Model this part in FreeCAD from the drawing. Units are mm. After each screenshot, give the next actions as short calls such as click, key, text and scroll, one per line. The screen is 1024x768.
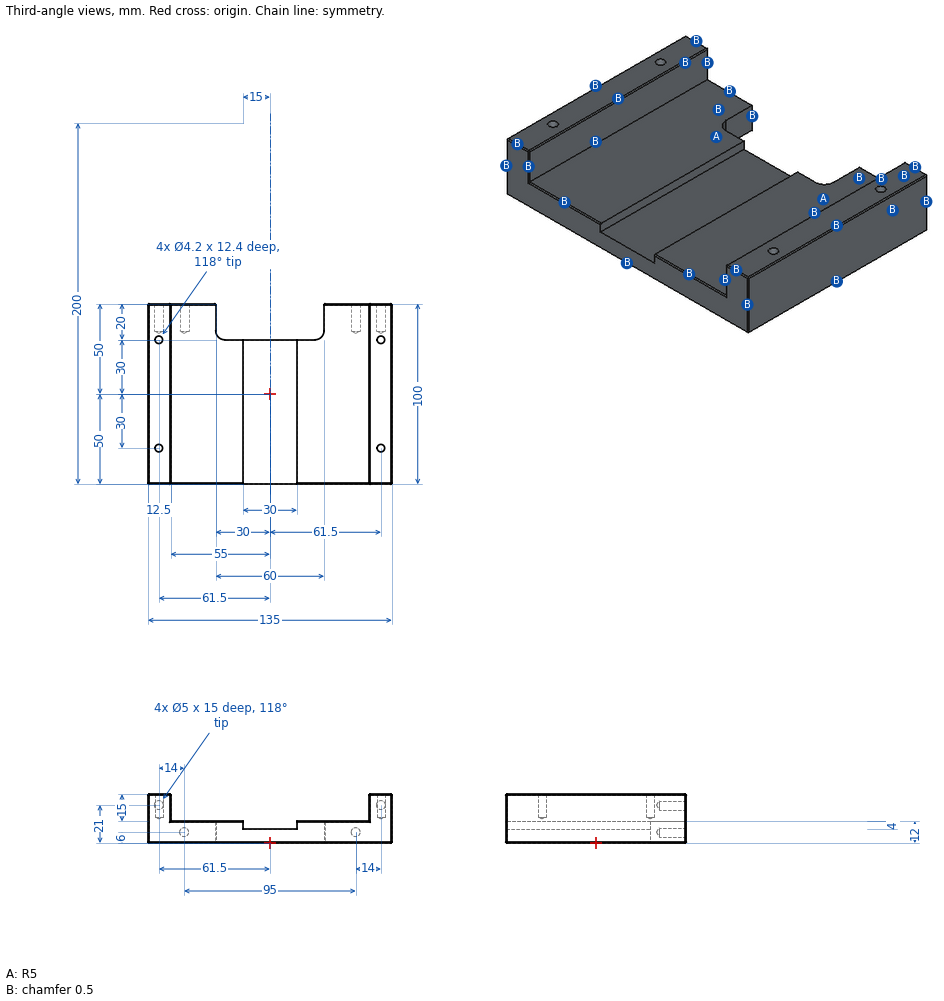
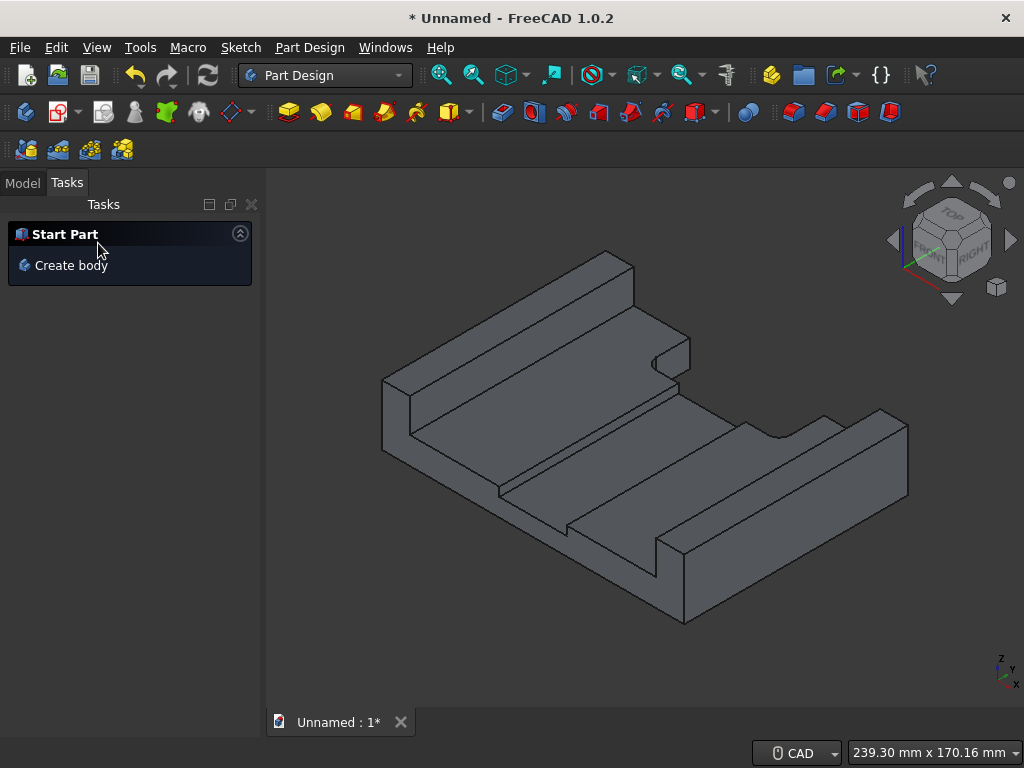
key(4)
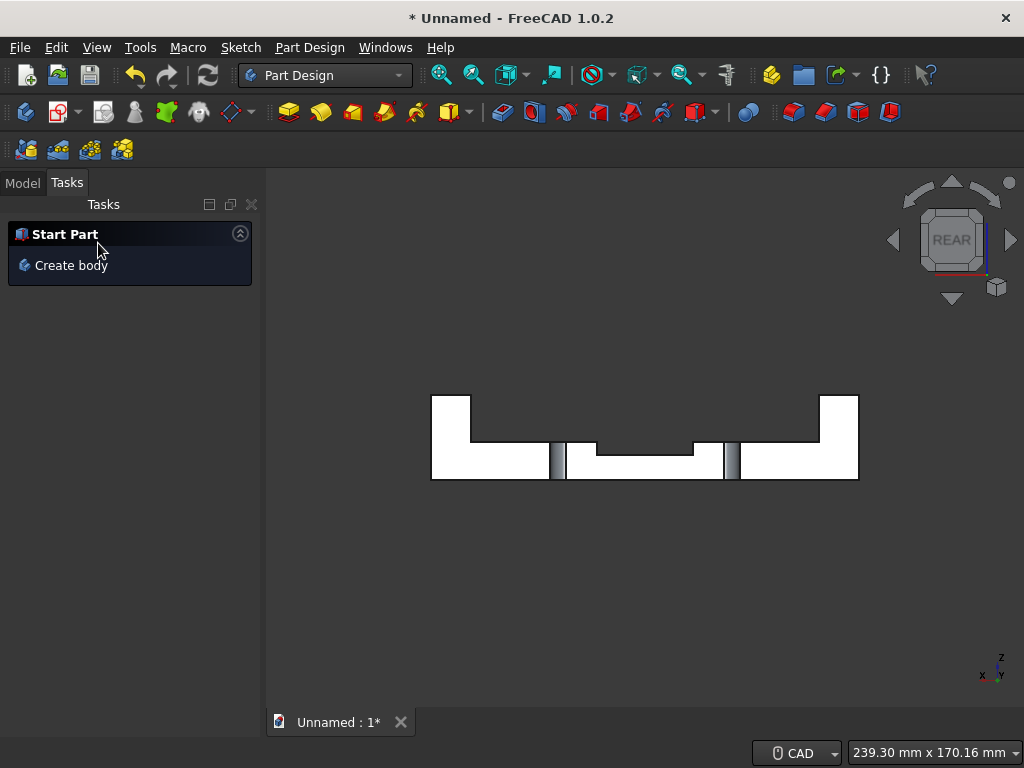
click(765, 461)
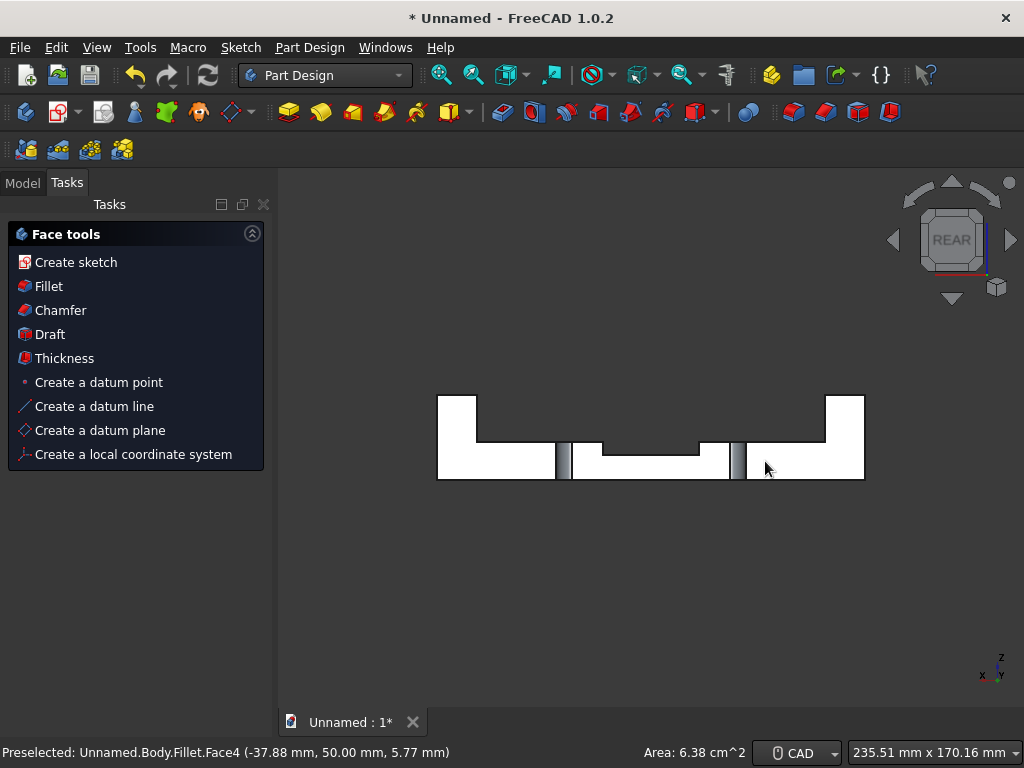
click(58, 112)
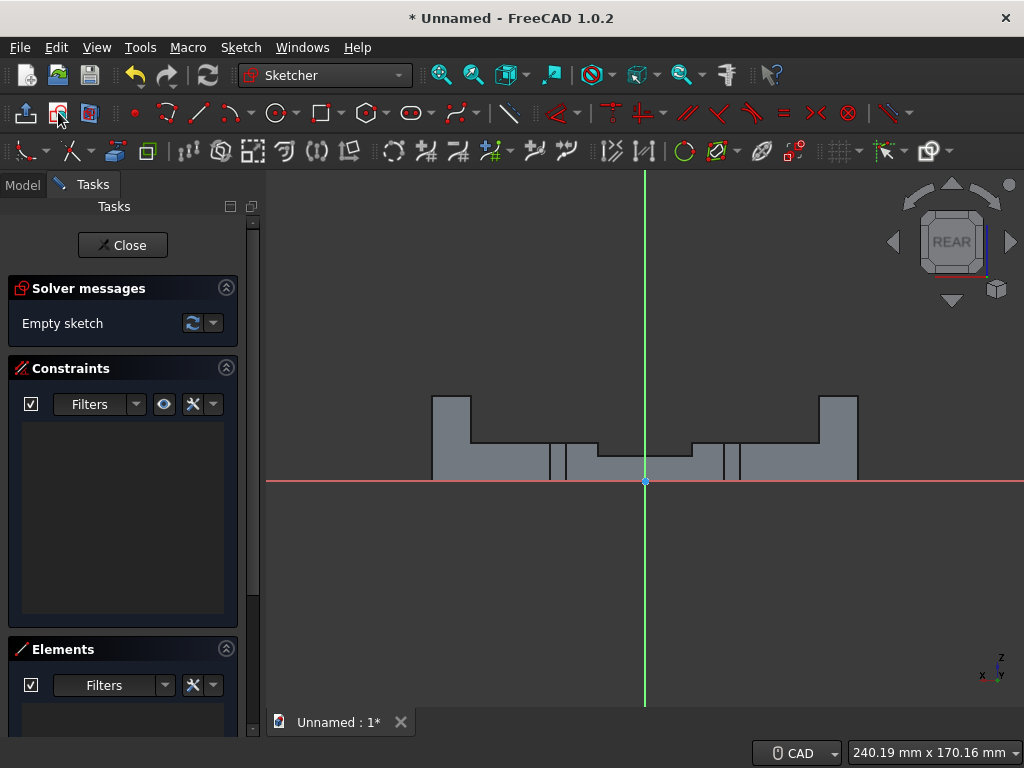
scroll(294, 414, down, 1)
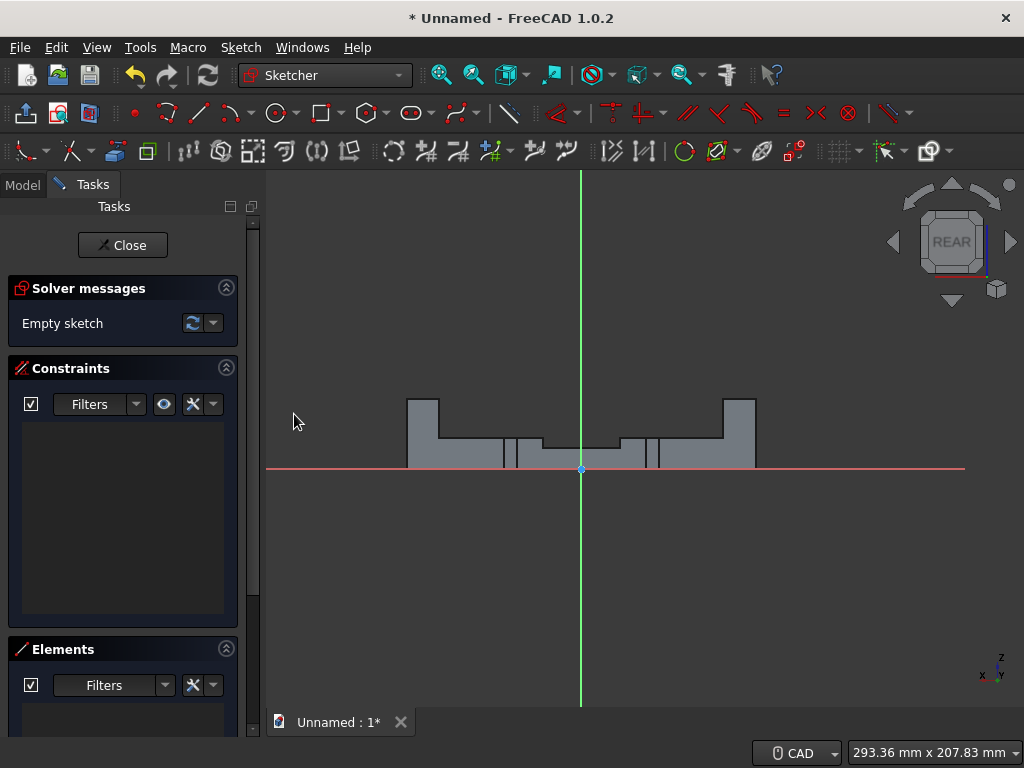
key(g)
key(c)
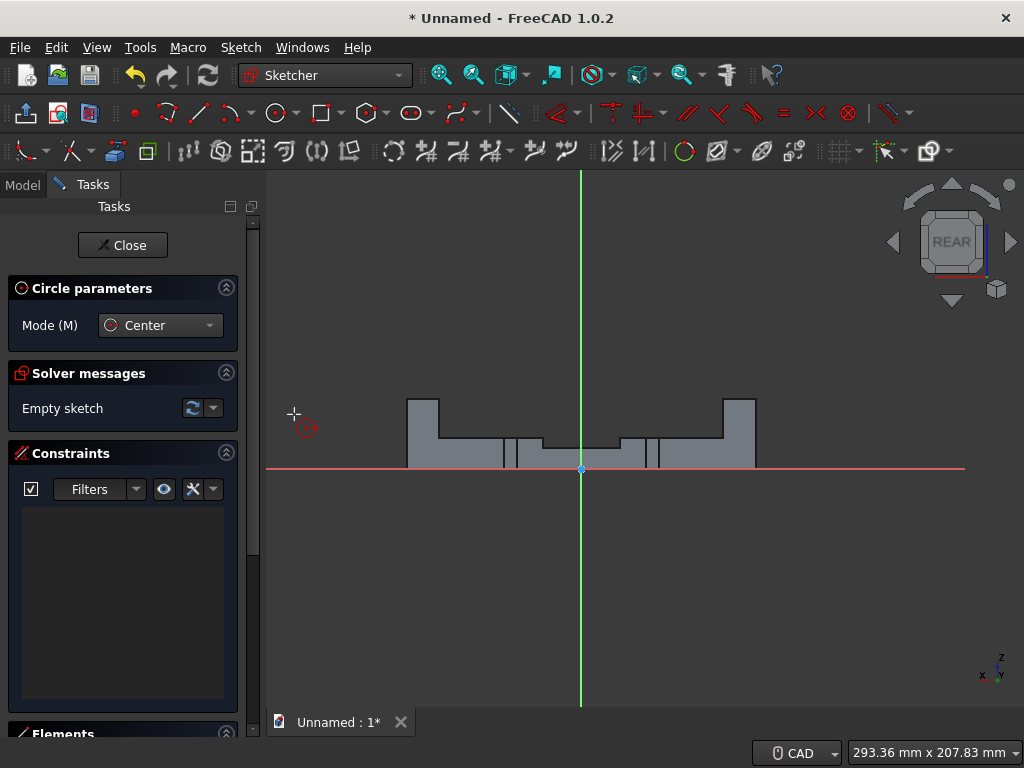
scroll(740, 415, up, 7)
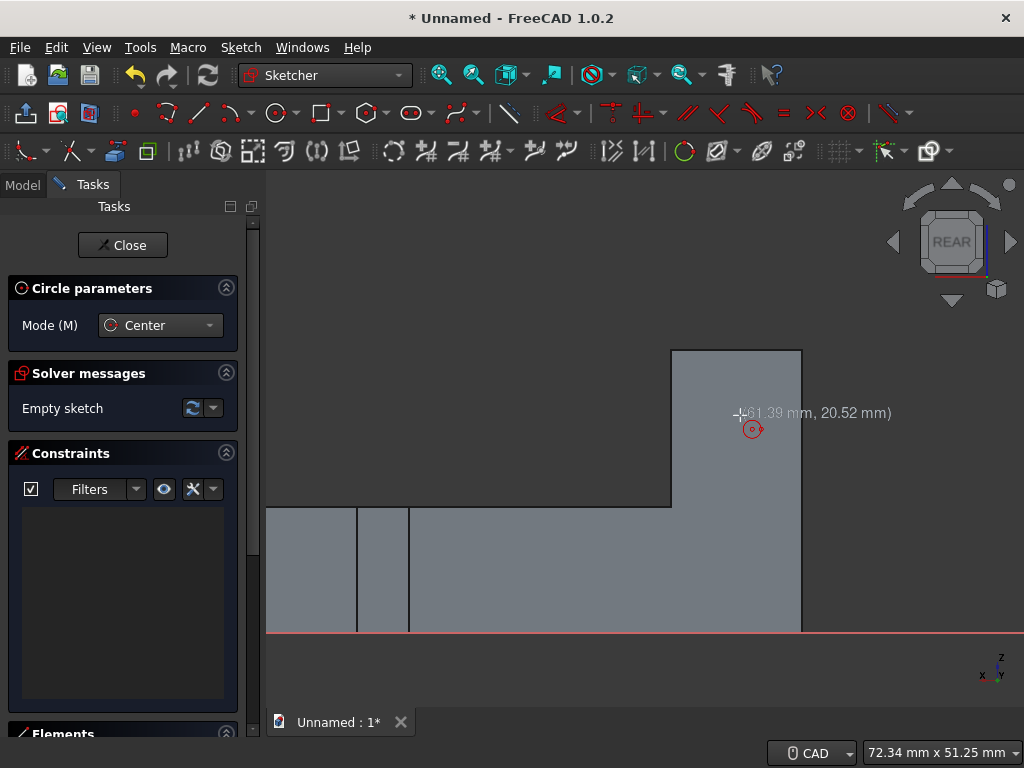
scroll(784, 408, down, 6)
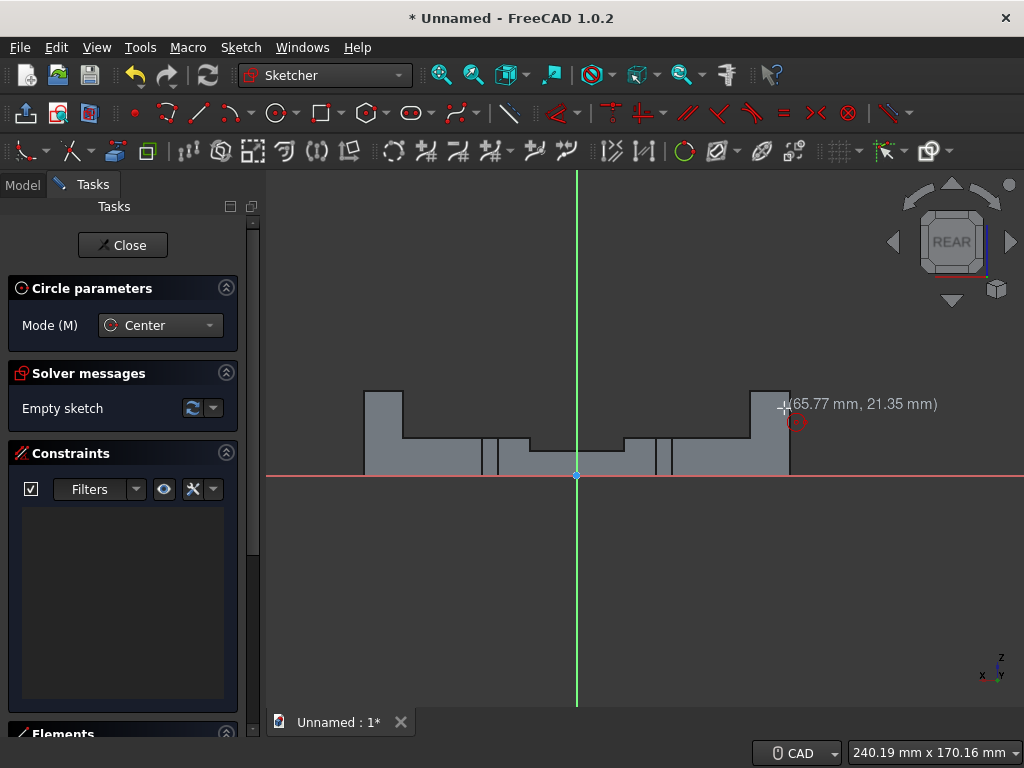
click(771, 410)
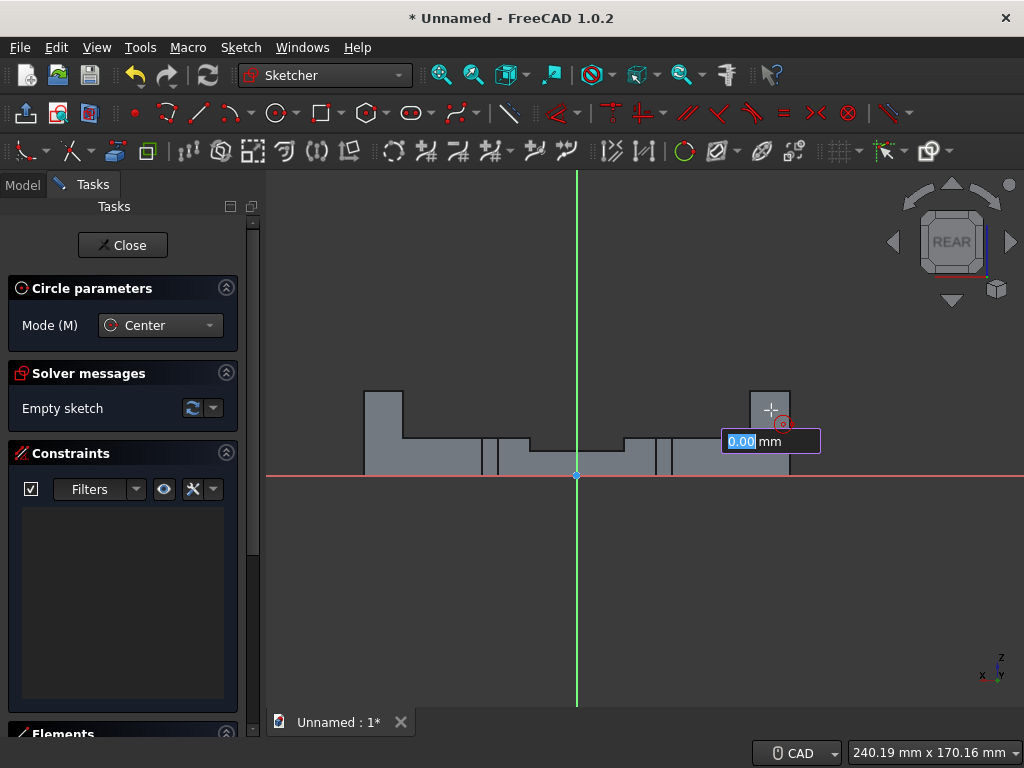
scroll(777, 404, up, 4)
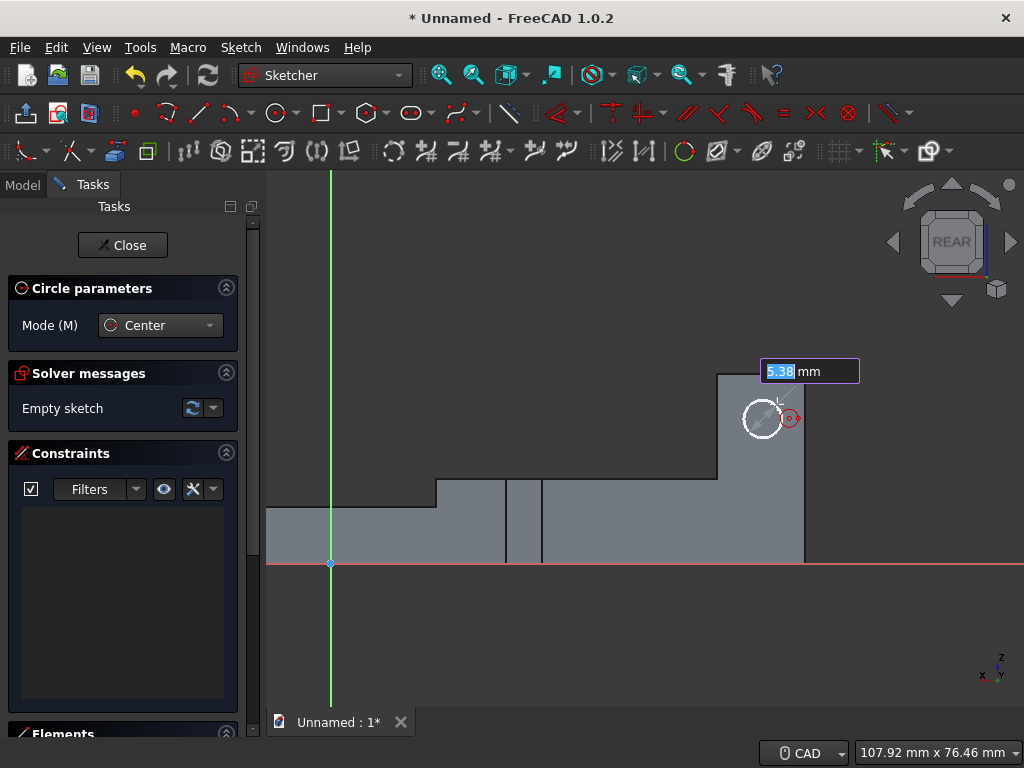
click(775, 404)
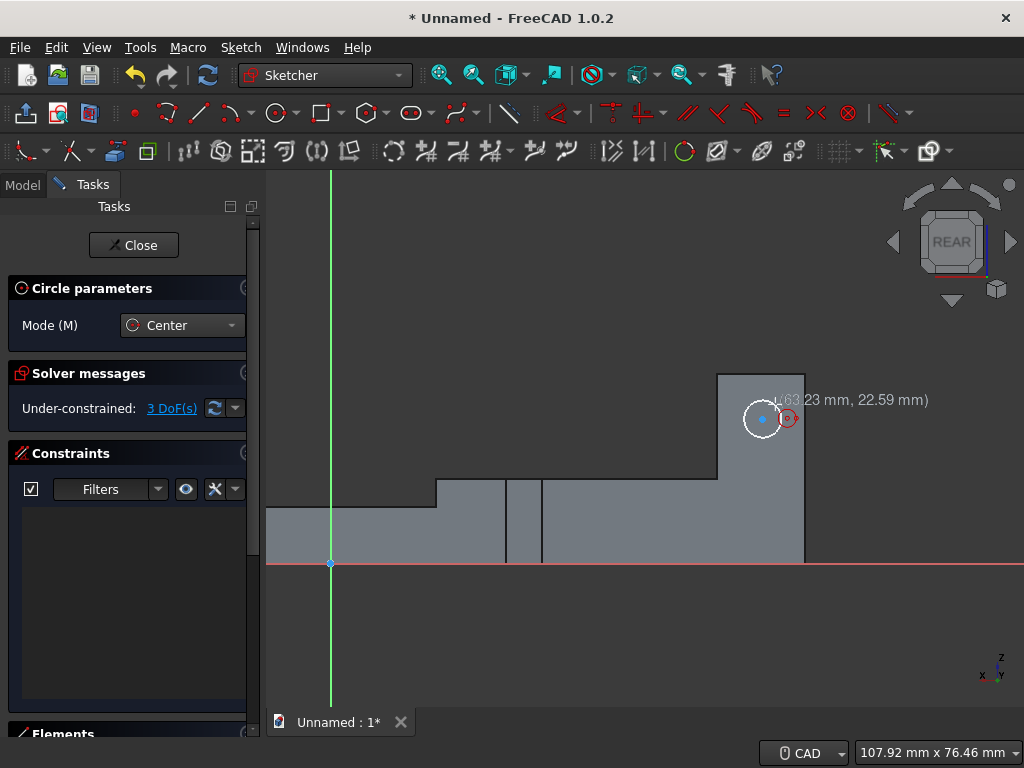
scroll(664, 522, up, 2)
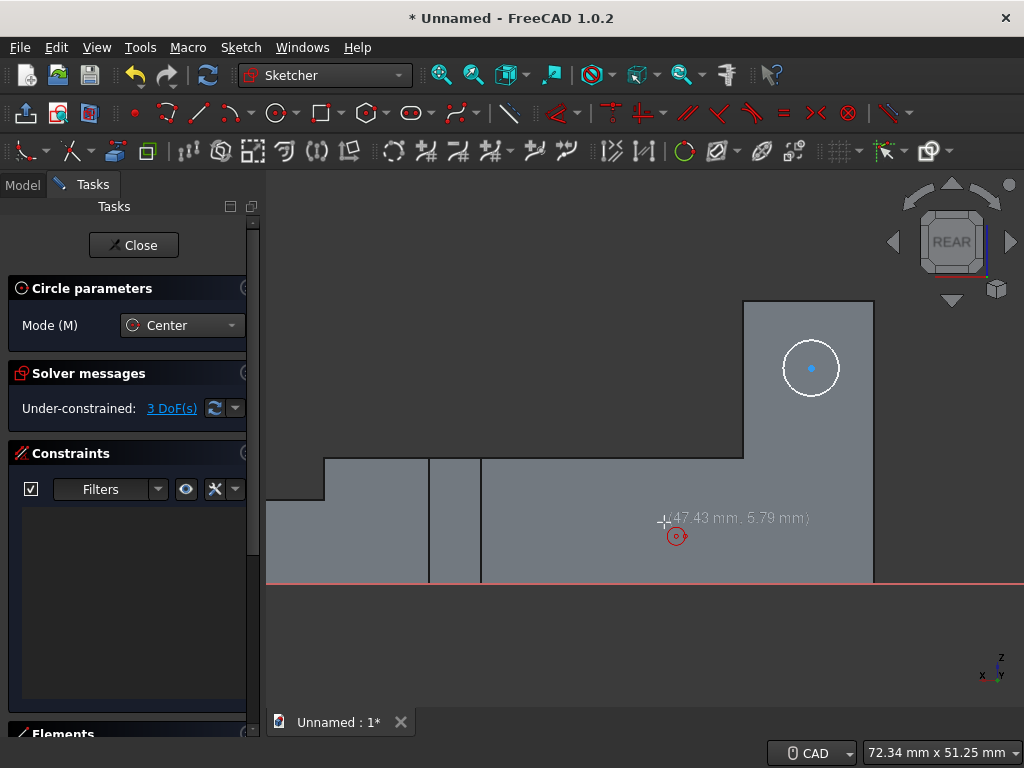
scroll(753, 429, down, 6)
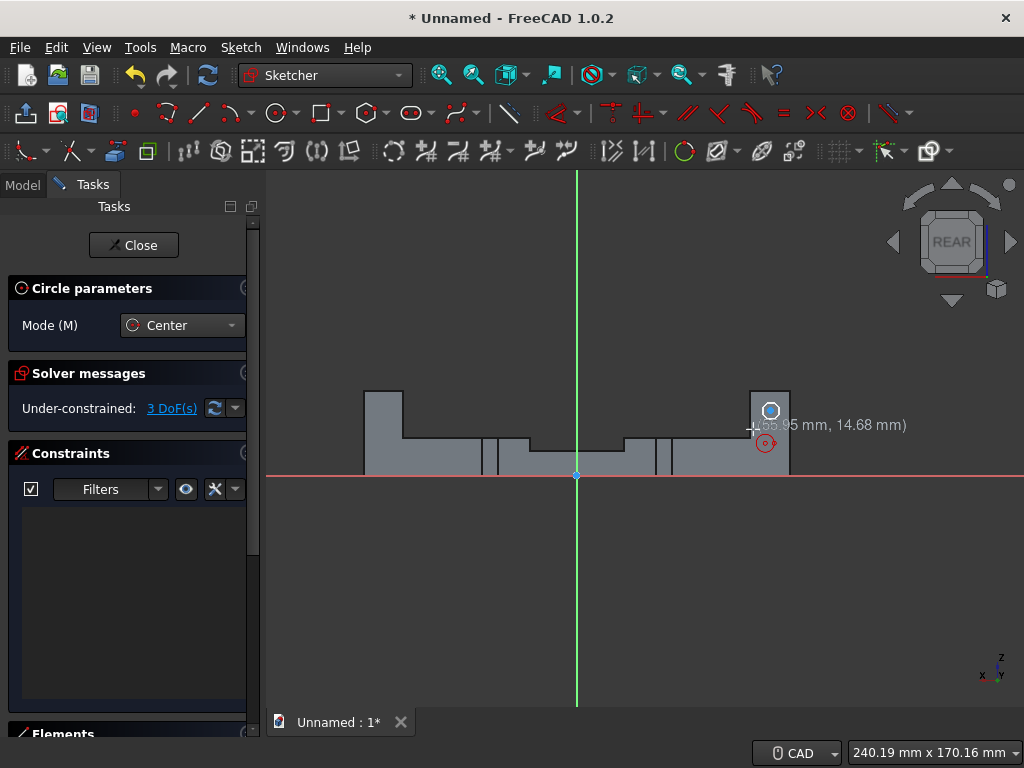
click(727, 457)